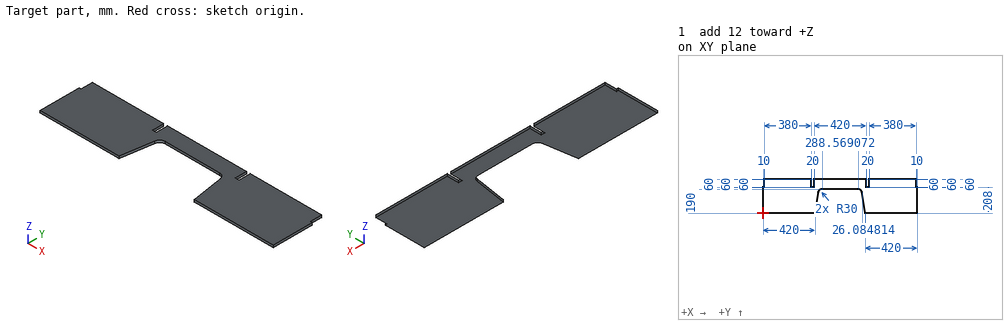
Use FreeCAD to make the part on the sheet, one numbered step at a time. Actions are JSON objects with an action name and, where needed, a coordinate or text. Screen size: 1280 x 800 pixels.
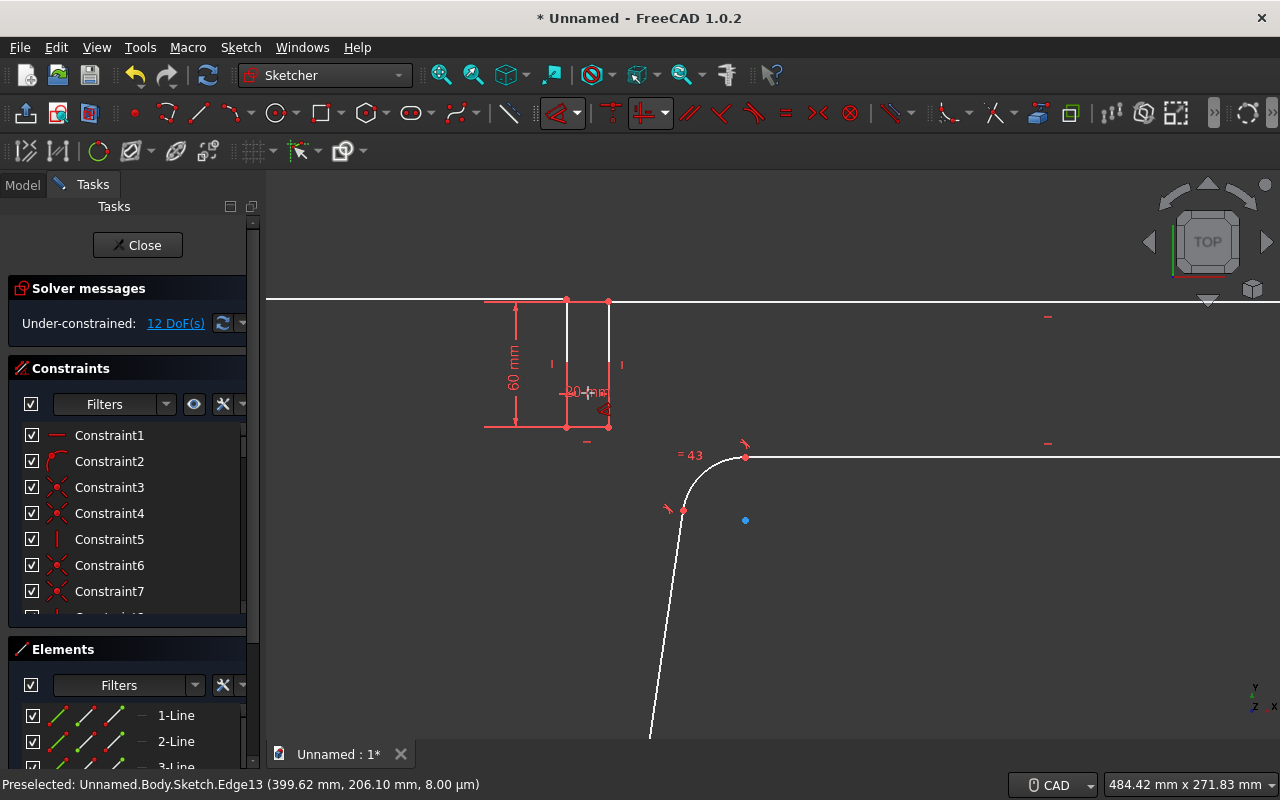
{"action": "left_click", "coordinate": [567, 389]}
{"action": "left_click", "coordinate": [533, 334]}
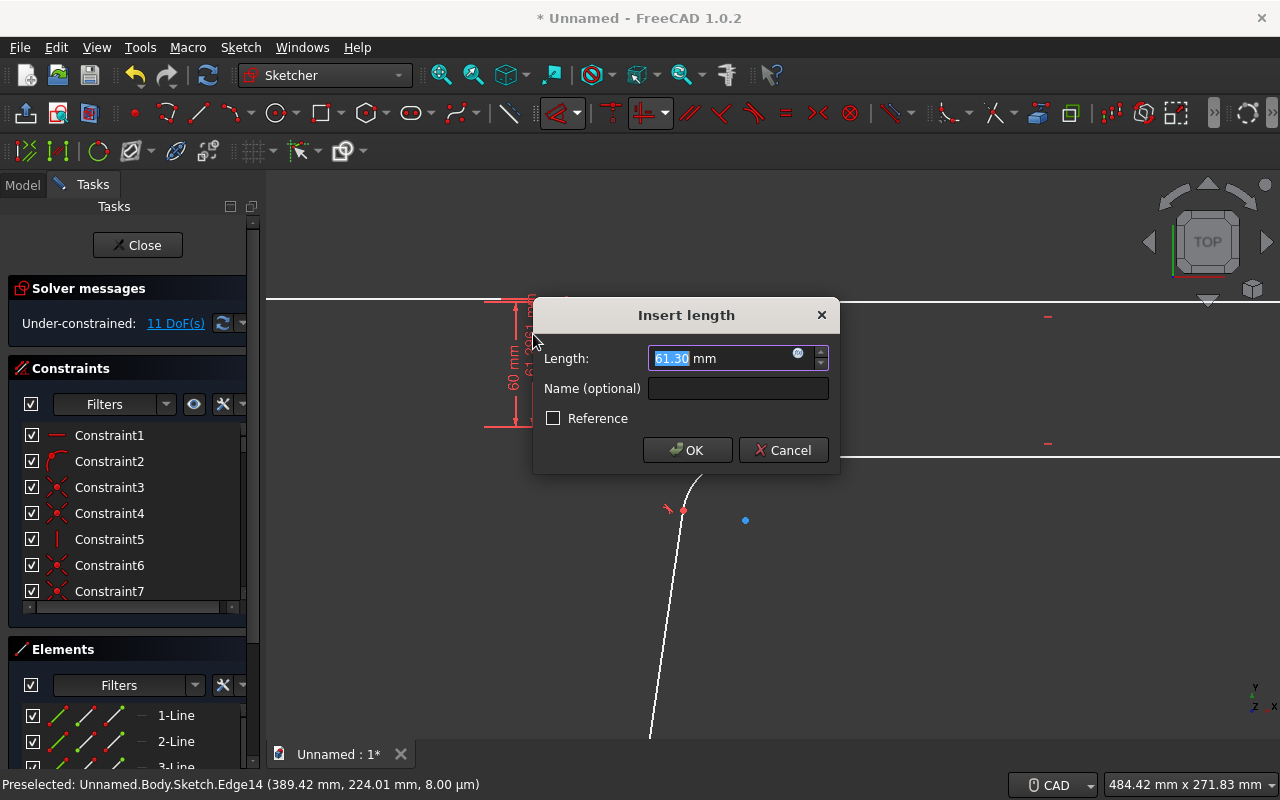
{"action": "type", "text": "60"}
{"action": "key", "text": "Return"}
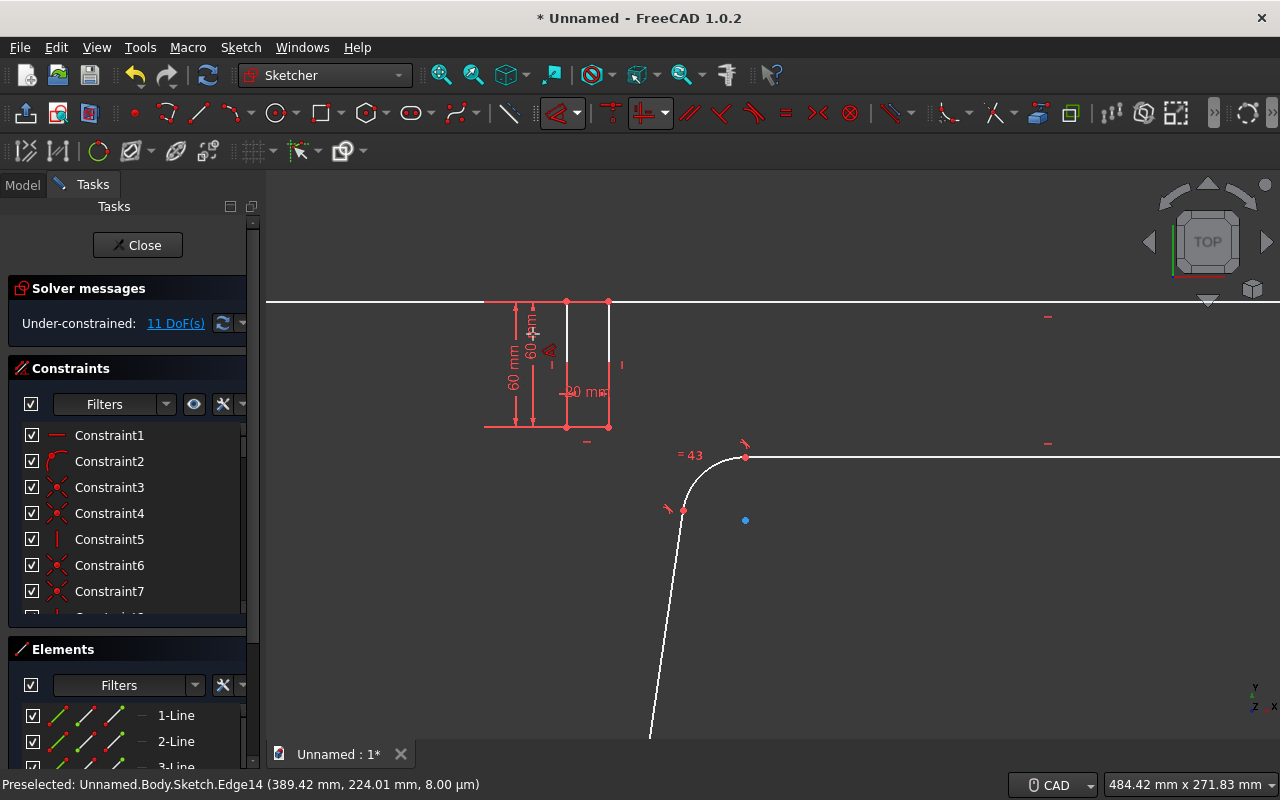
{"action": "scroll", "coordinate": [592, 414], "scroll_direction": "down", "scroll_amount": 7}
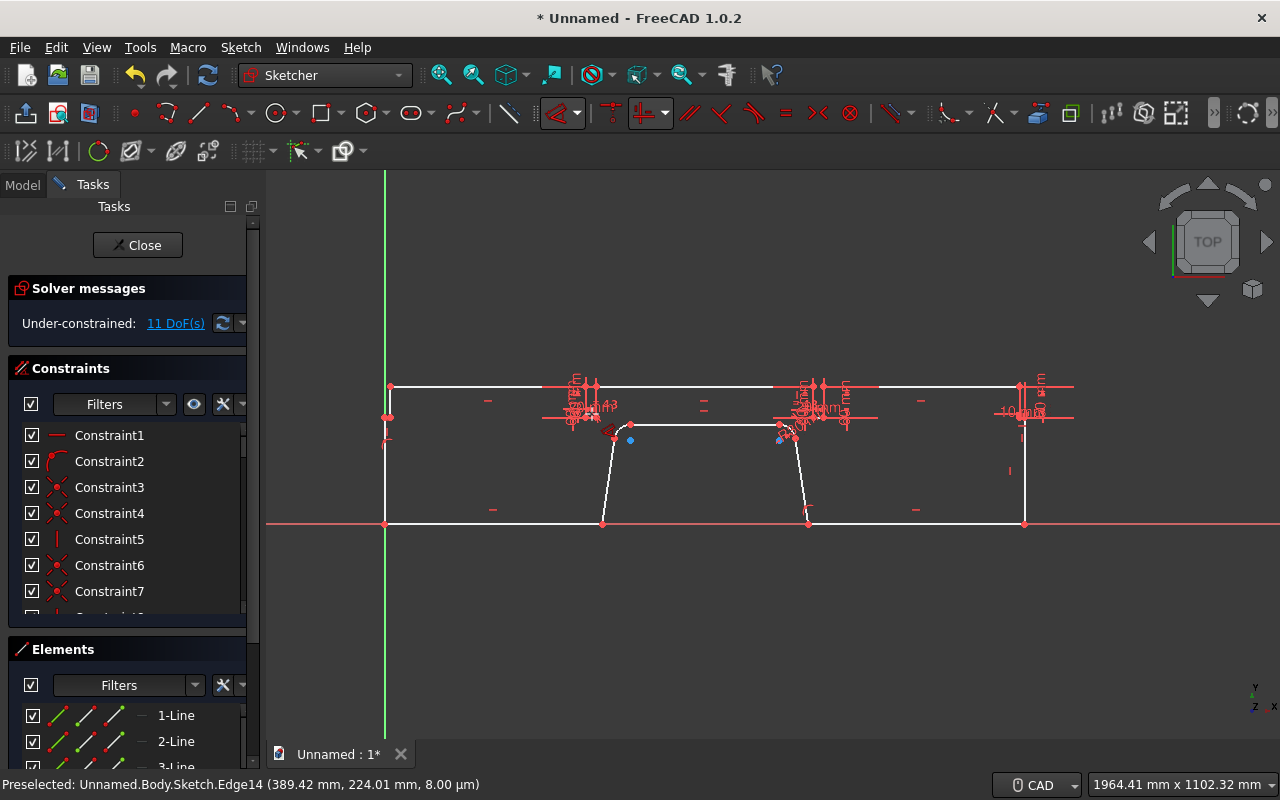
{"action": "scroll", "coordinate": [390, 396], "scroll_direction": "up", "scroll_amount": 5}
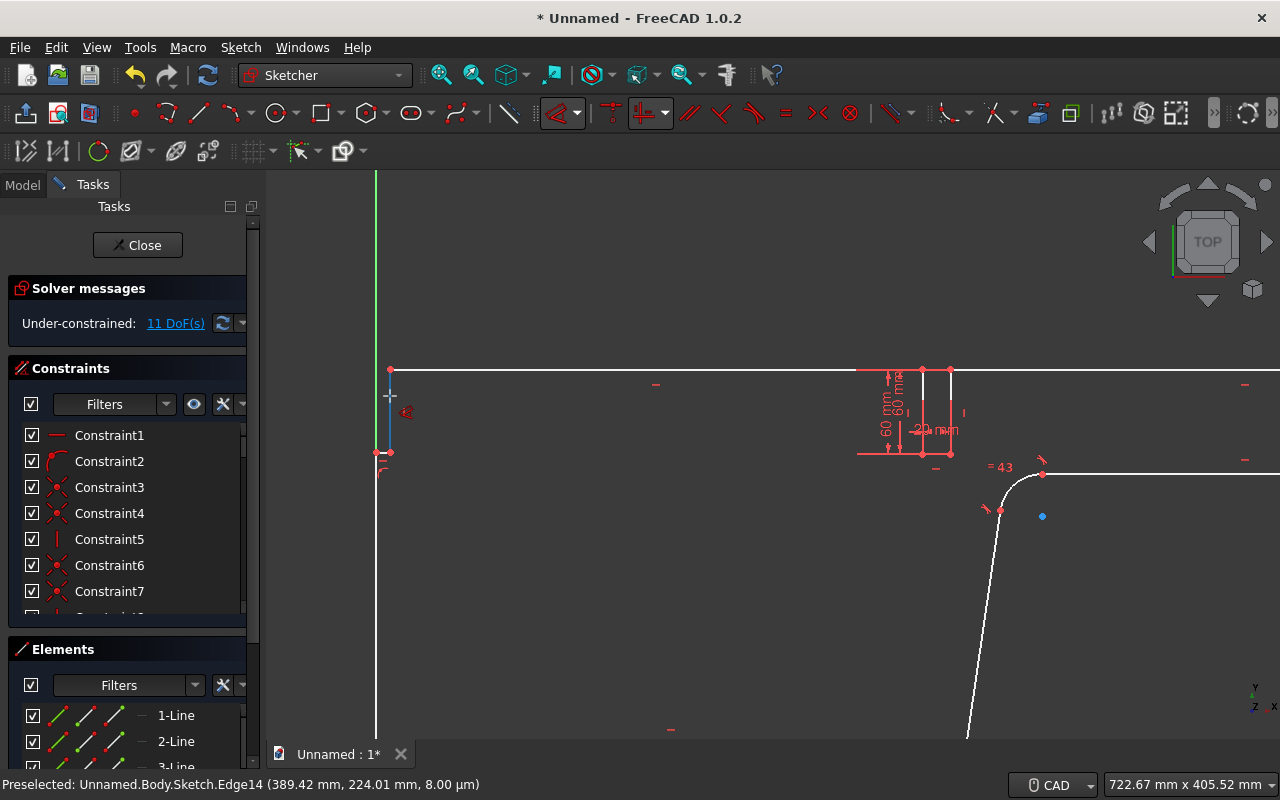
{"action": "left_click", "coordinate": [390, 395]}
{"action": "left_click", "coordinate": [356, 411]}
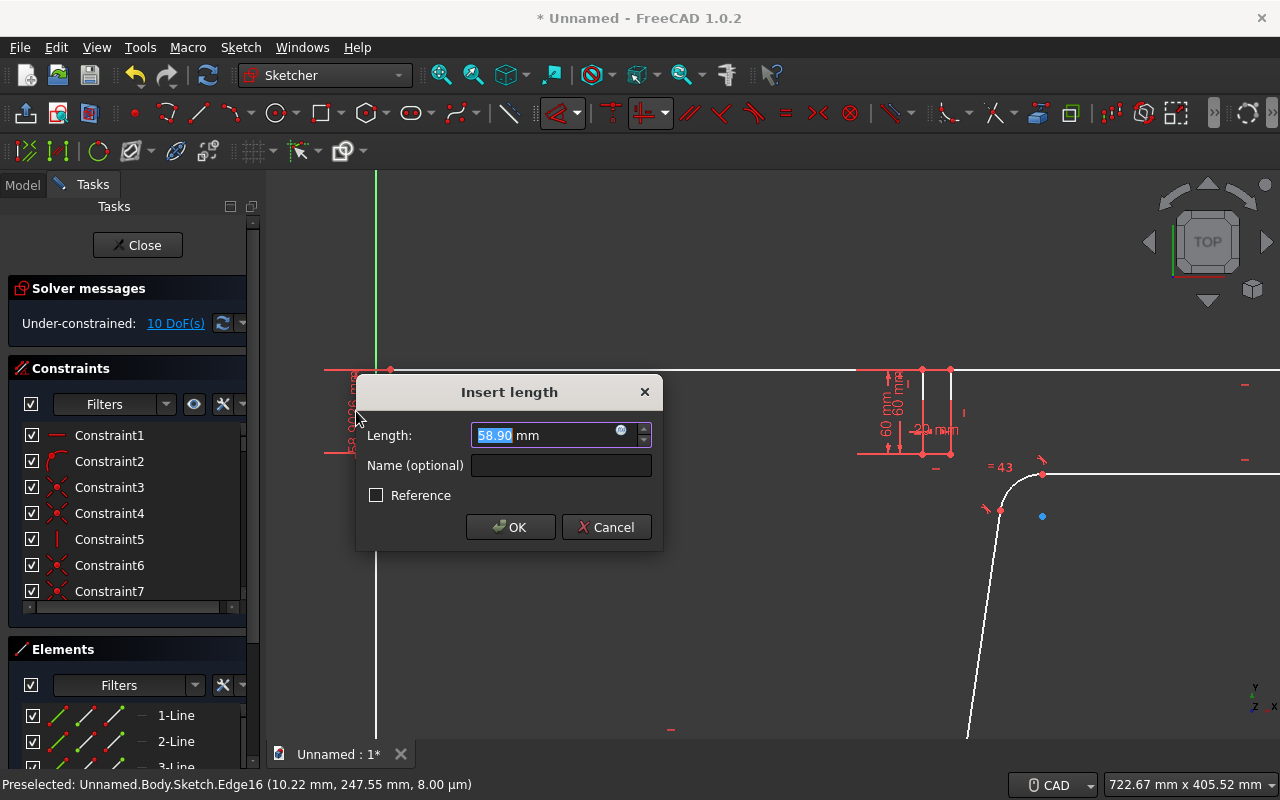
{"action": "type", "text": "60"}
{"action": "key", "text": "Return"}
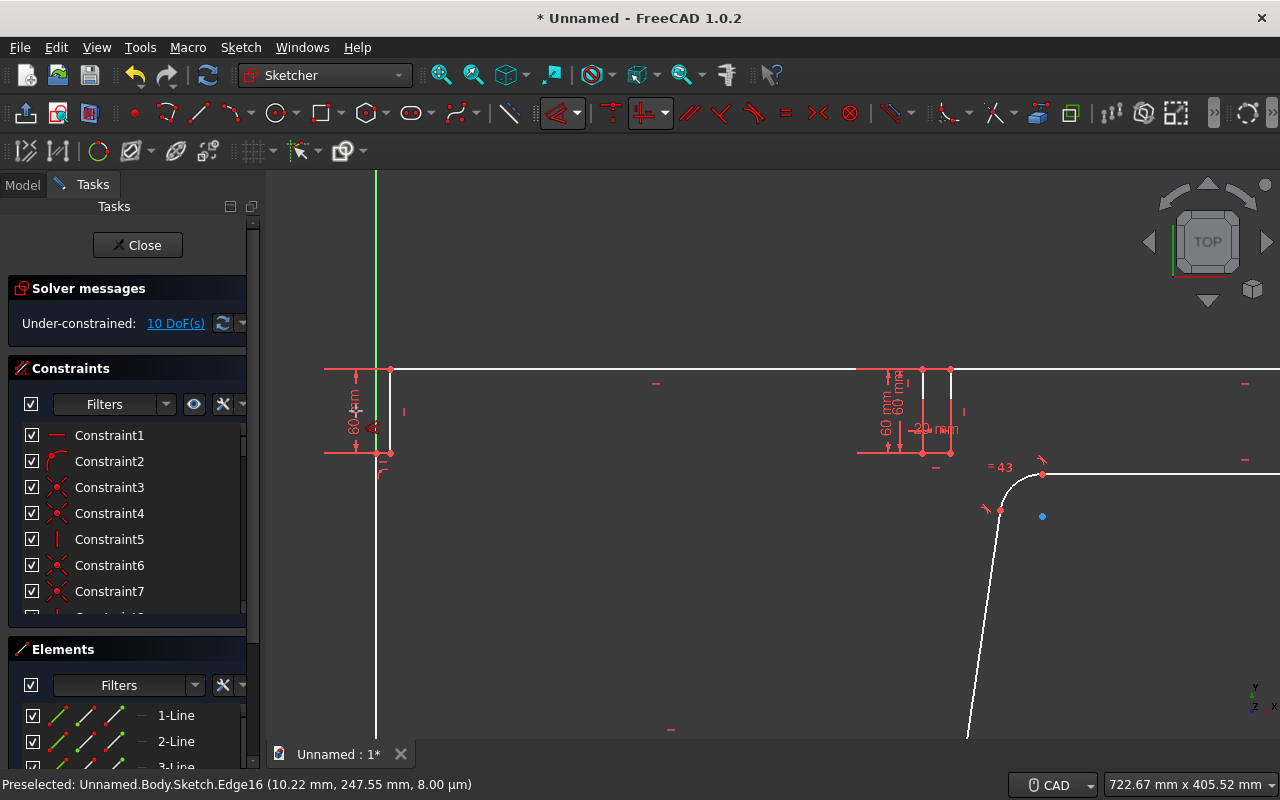
{"action": "scroll", "coordinate": [383, 453], "scroll_direction": "up", "scroll_amount": 6}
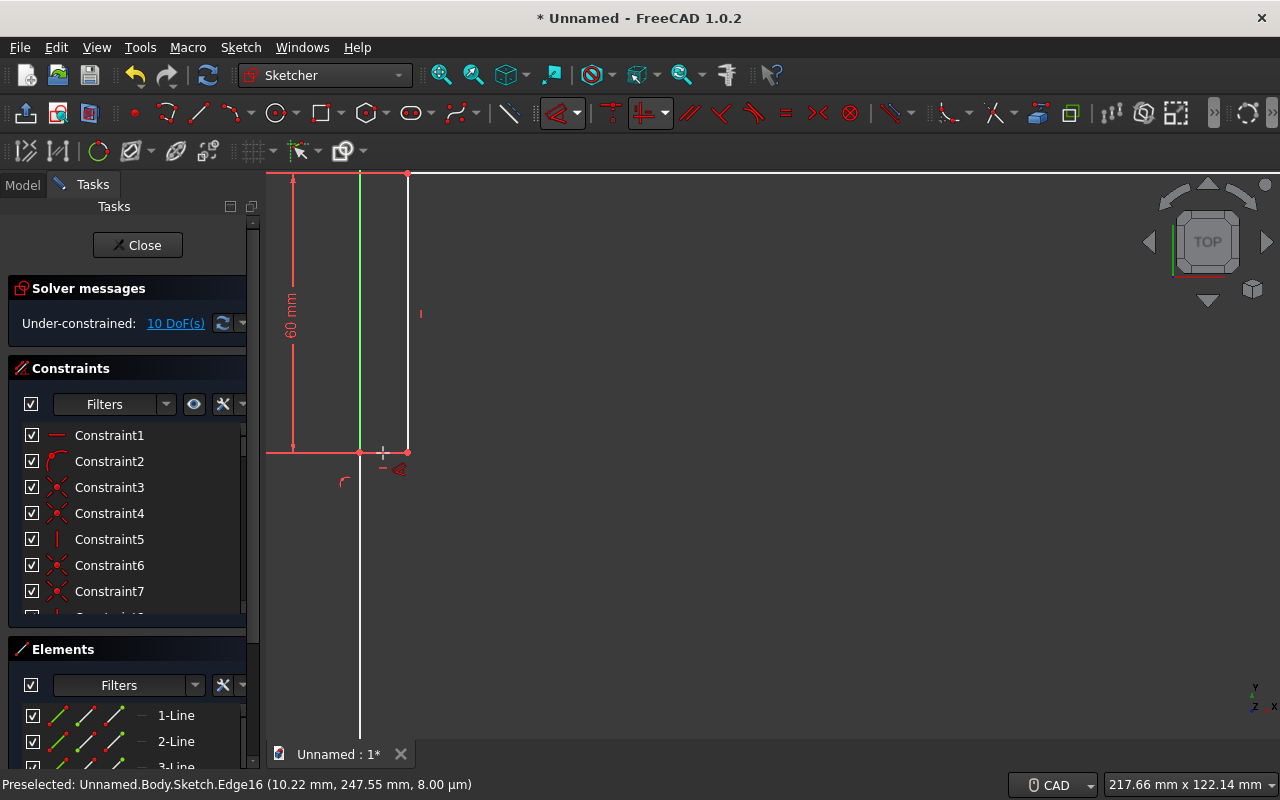
{"action": "left_click", "coordinate": [384, 453]}
{"action": "left_click", "coordinate": [384, 419]}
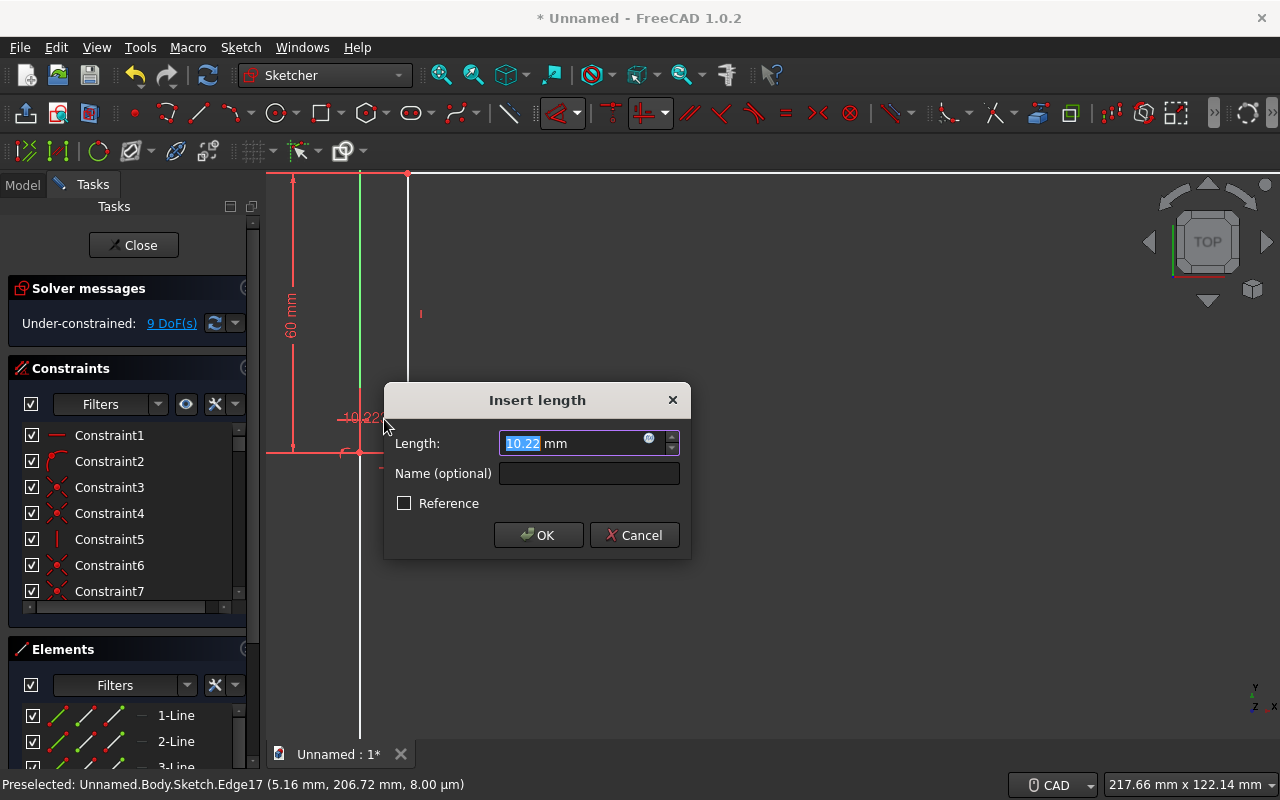
{"action": "type", "text": "10"}
{"action": "key", "text": "Return"}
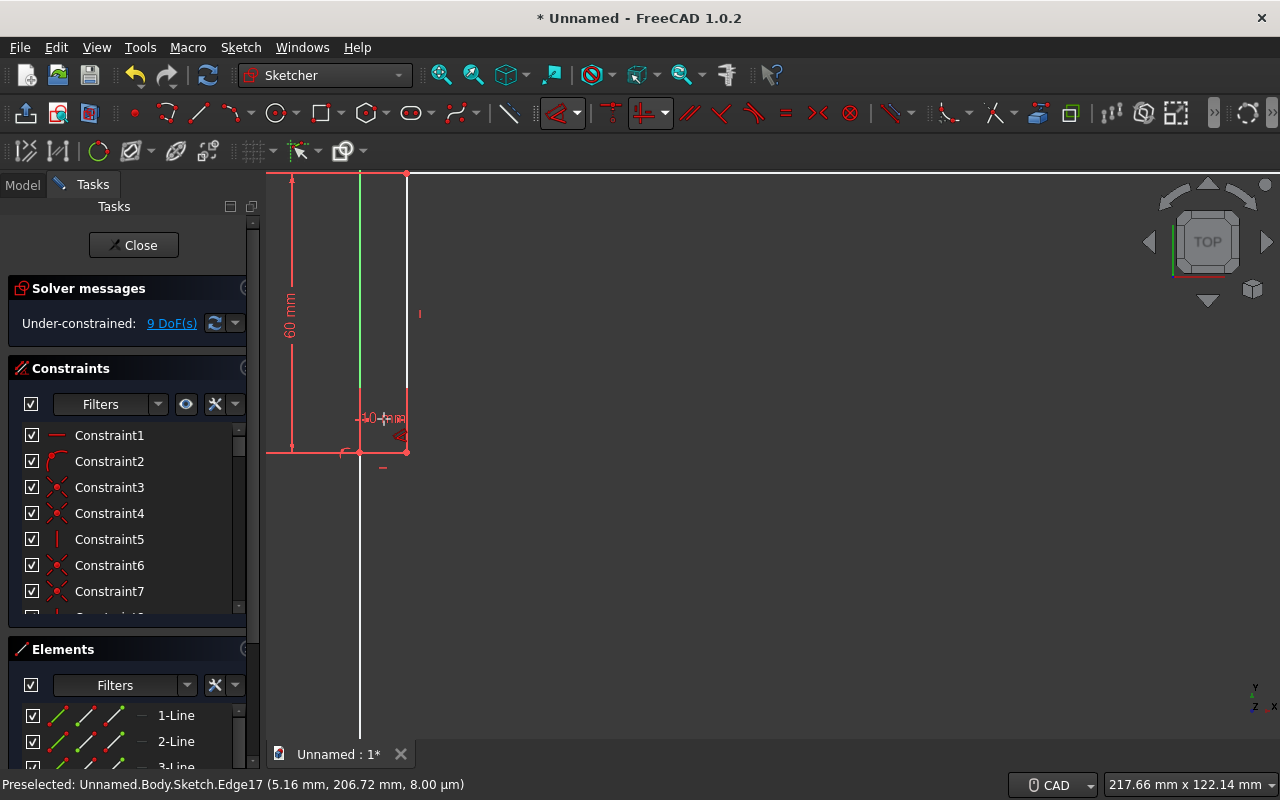
{"action": "scroll", "coordinate": [388, 412], "scroll_direction": "down", "scroll_amount": 11}